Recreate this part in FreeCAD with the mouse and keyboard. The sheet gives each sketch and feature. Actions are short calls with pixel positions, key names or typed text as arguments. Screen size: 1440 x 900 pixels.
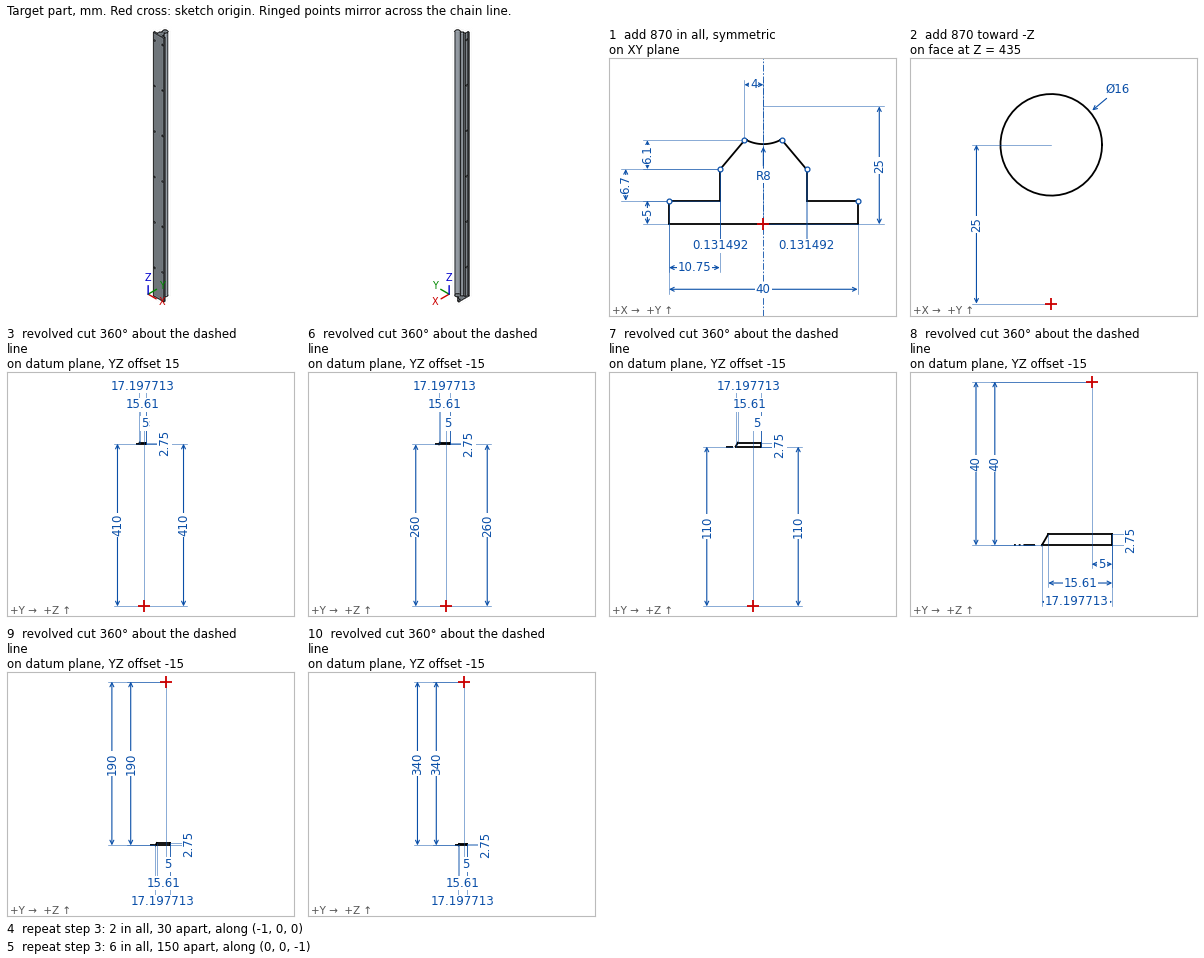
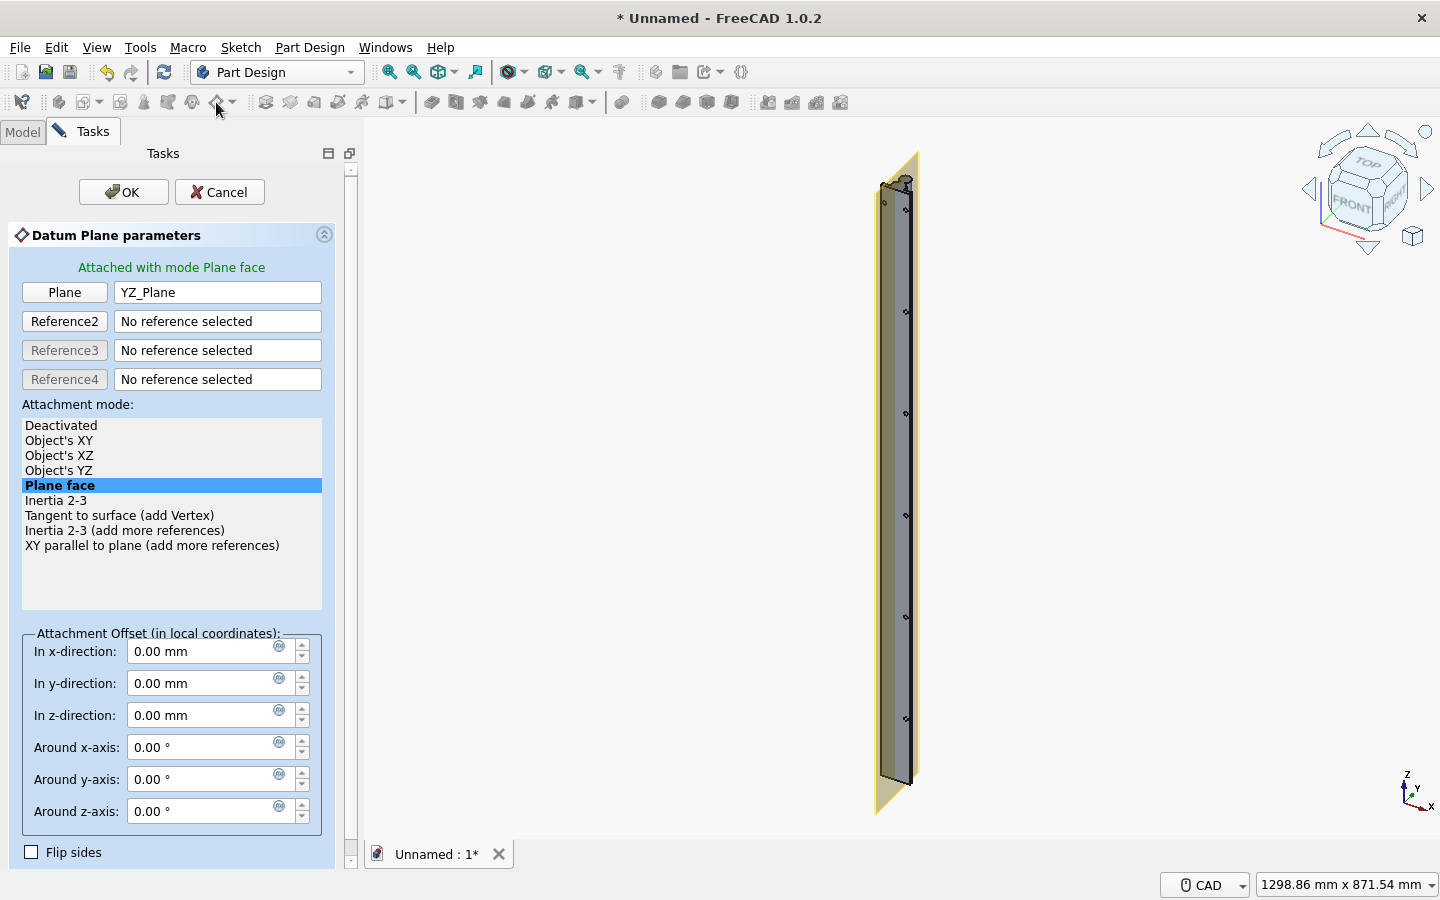
triple_click(210, 715)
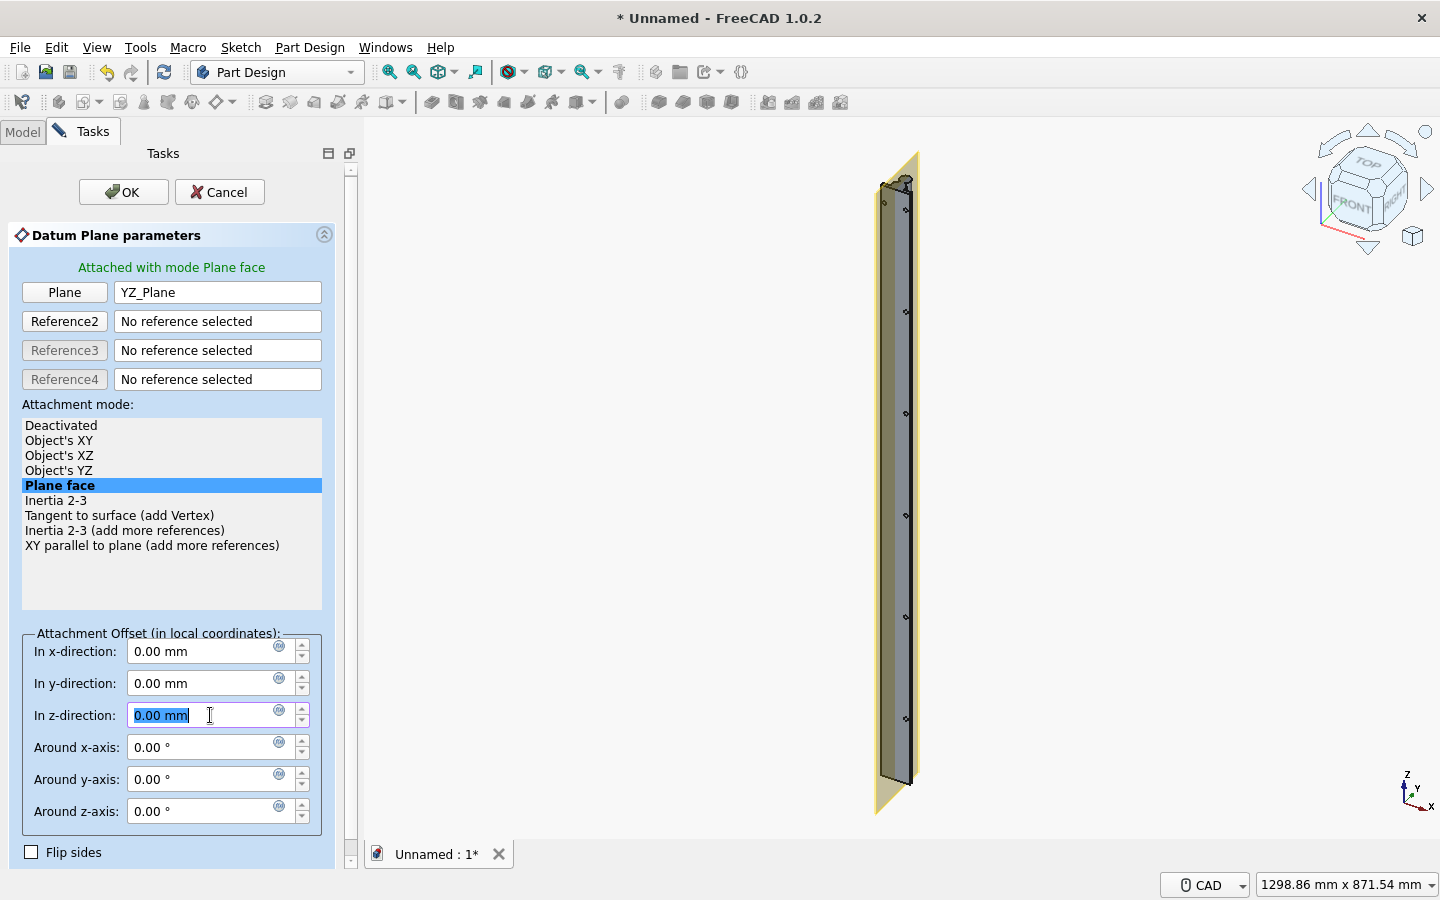
text(-15)
key(Tab)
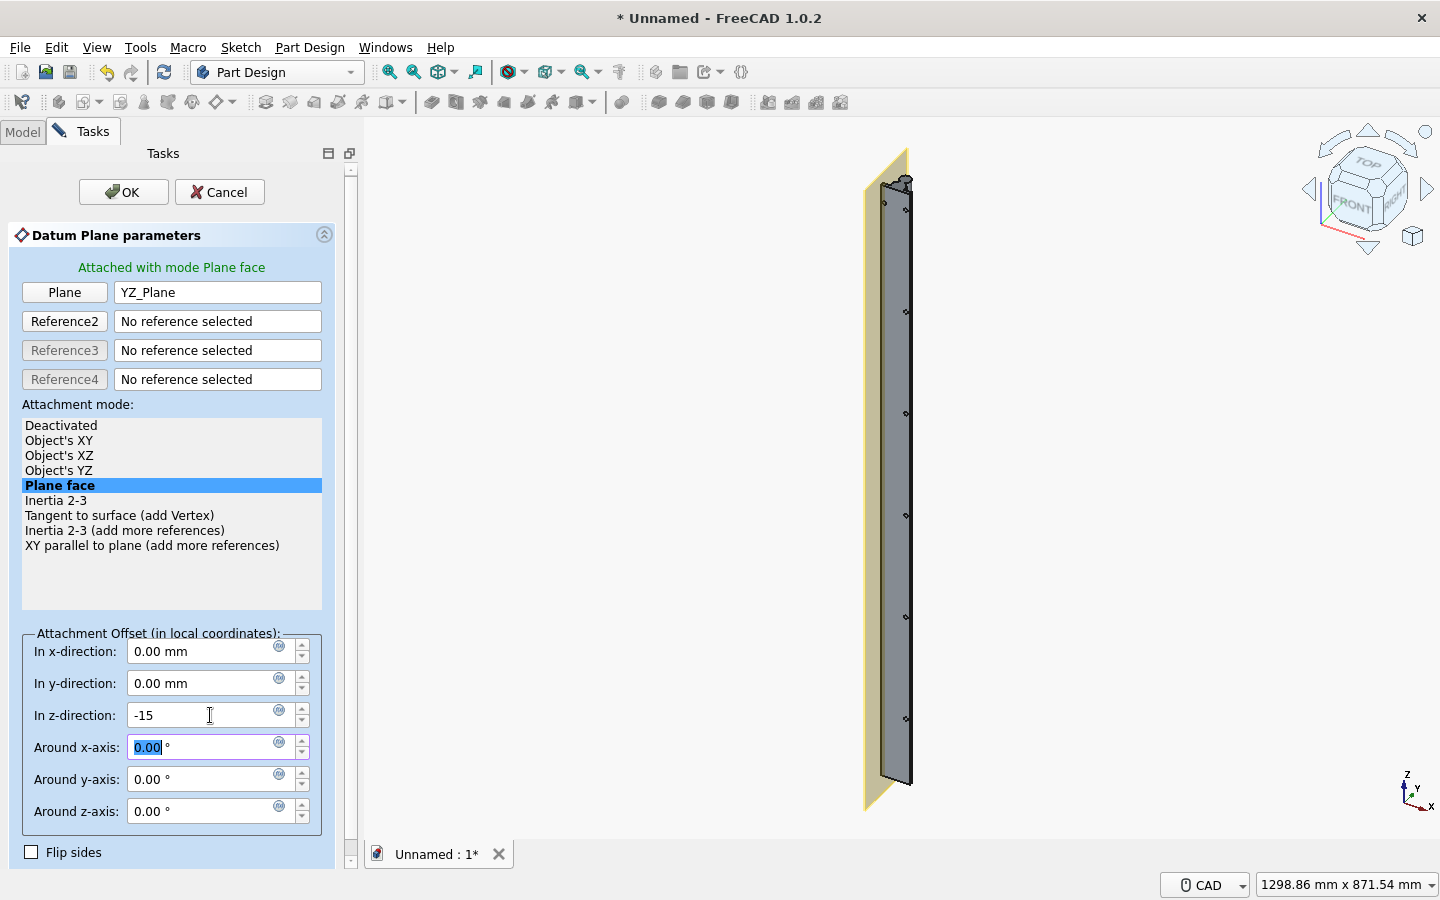
click(124, 192)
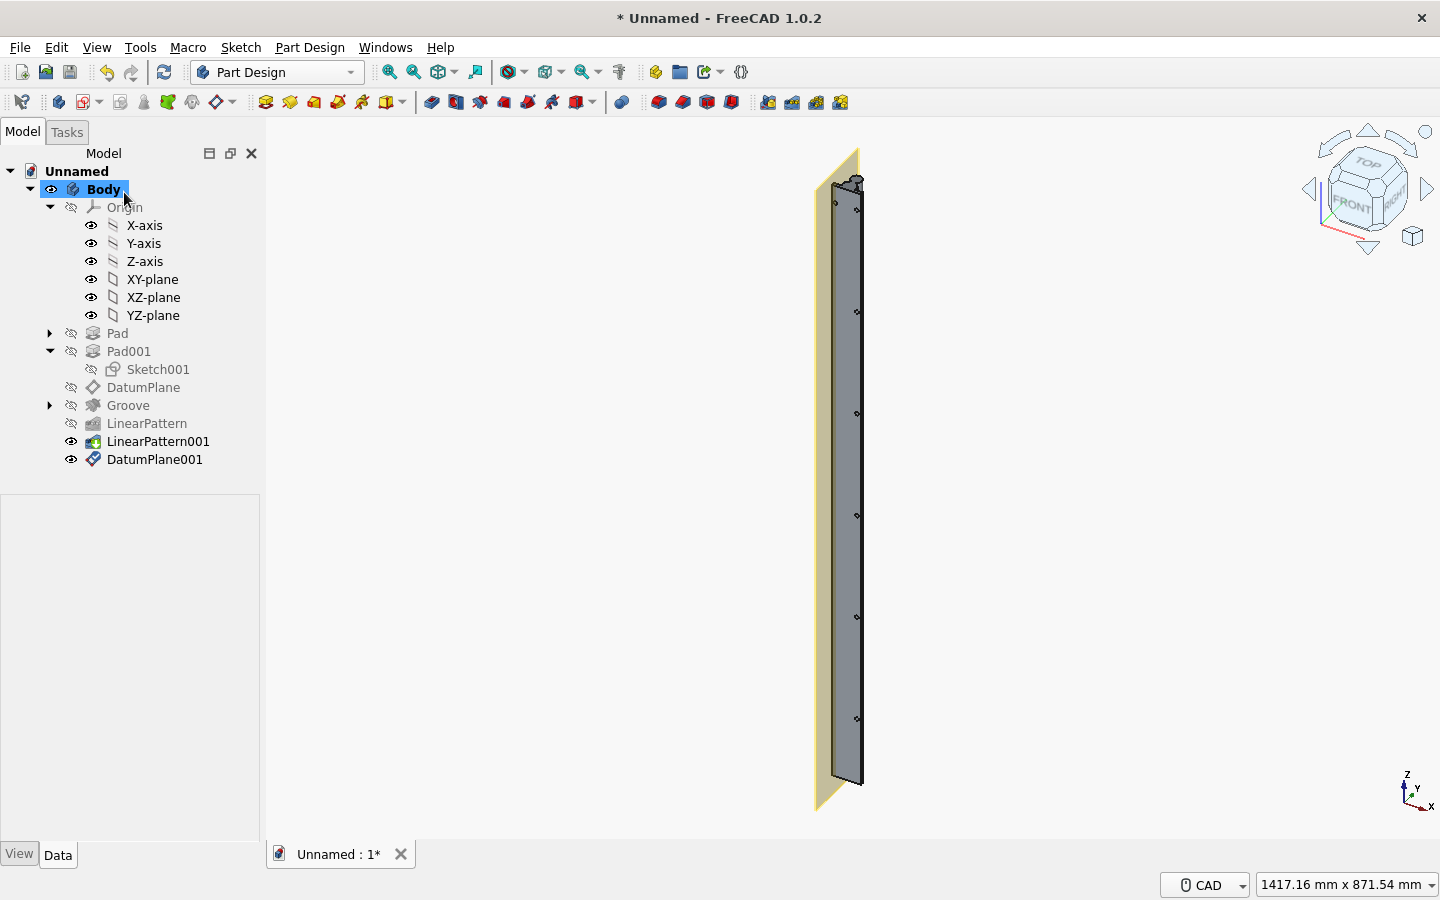
click(116, 459)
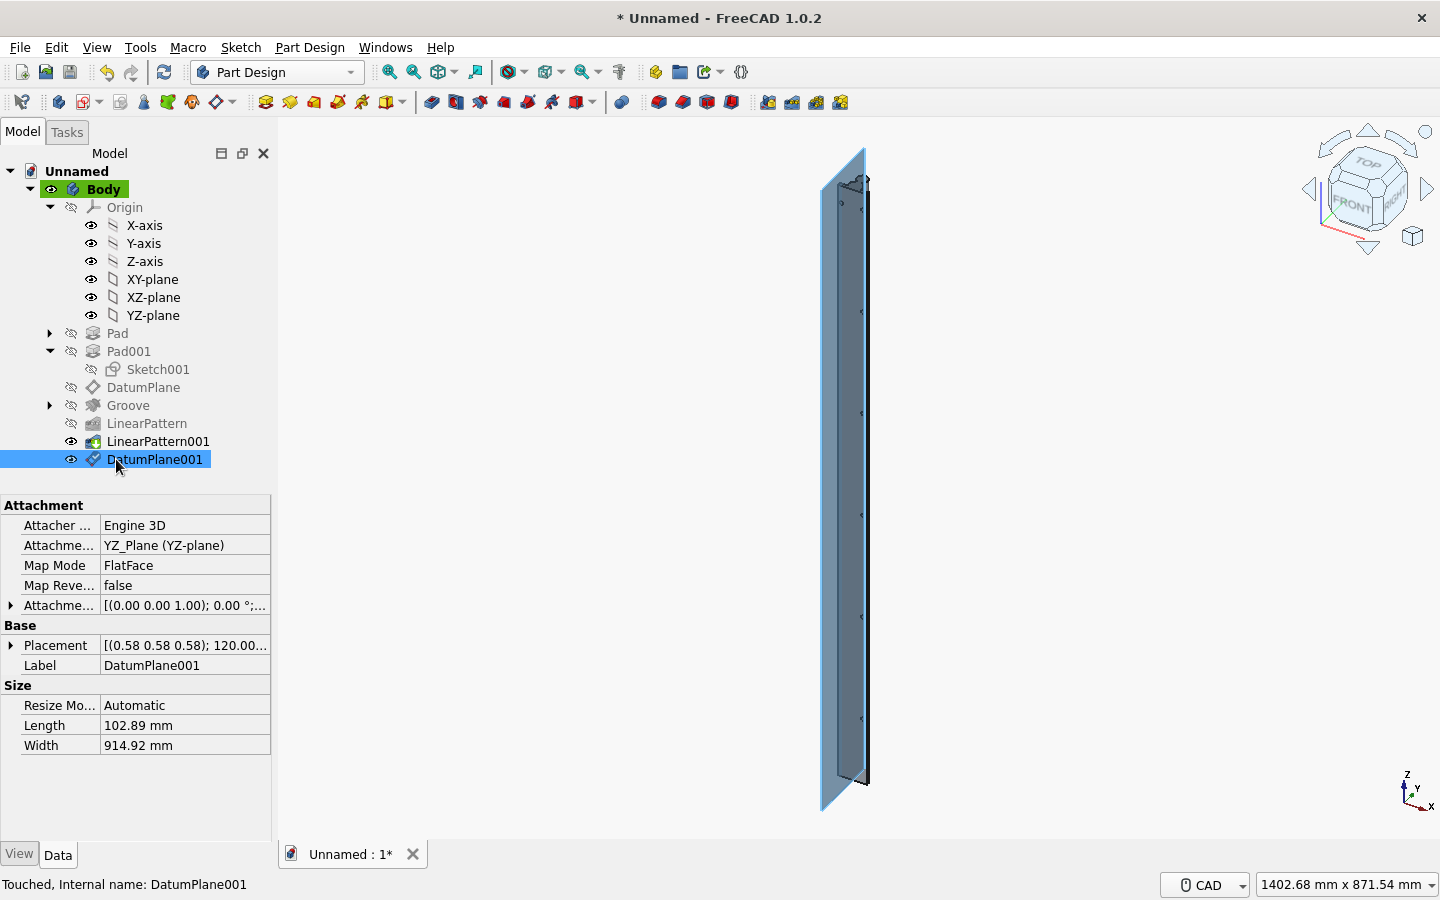
click(84, 102)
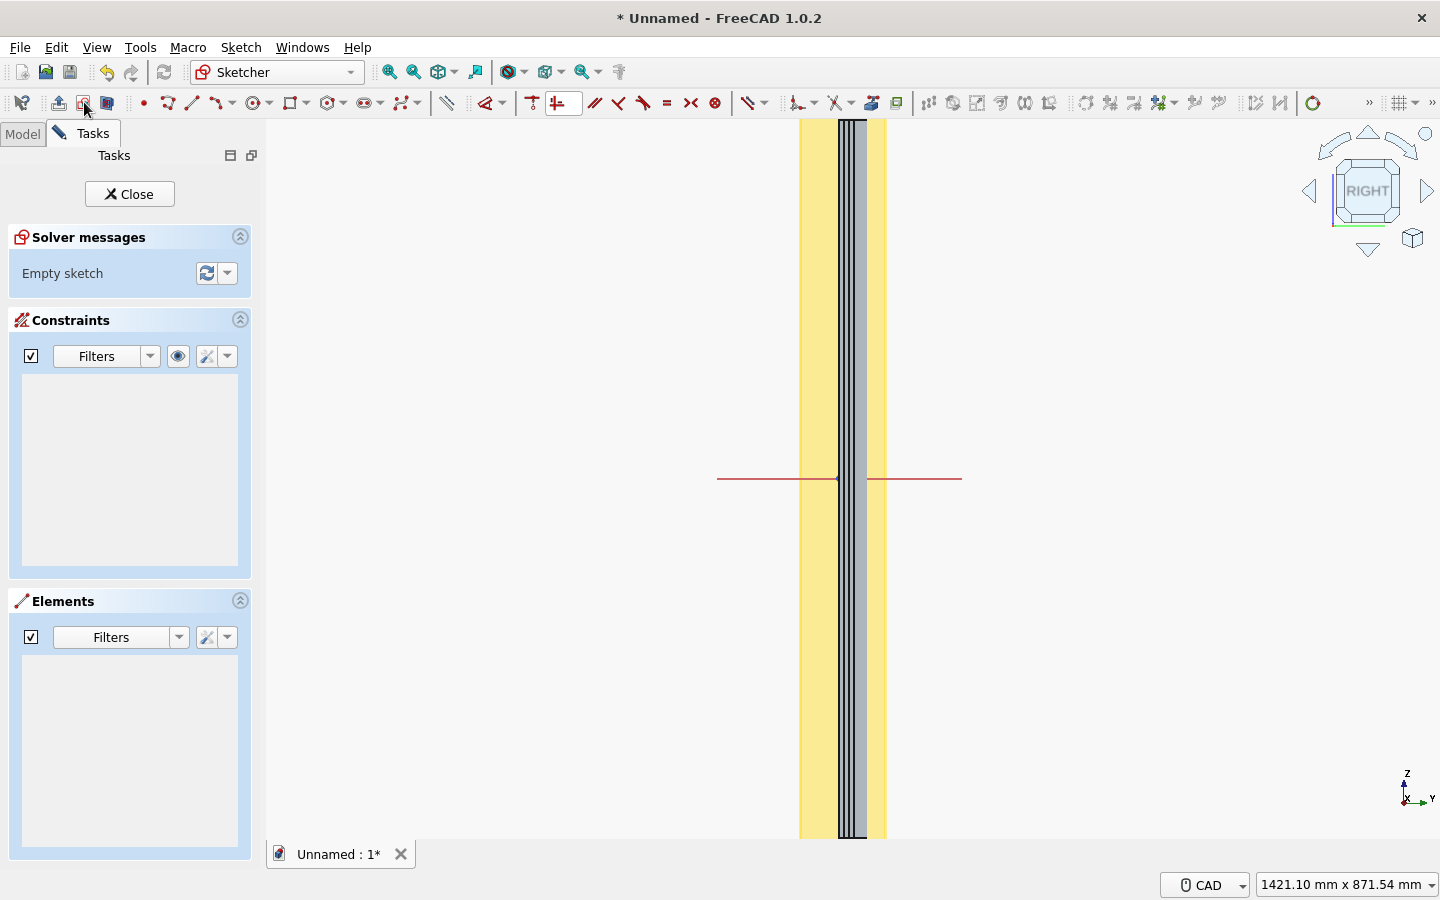
click(108, 104)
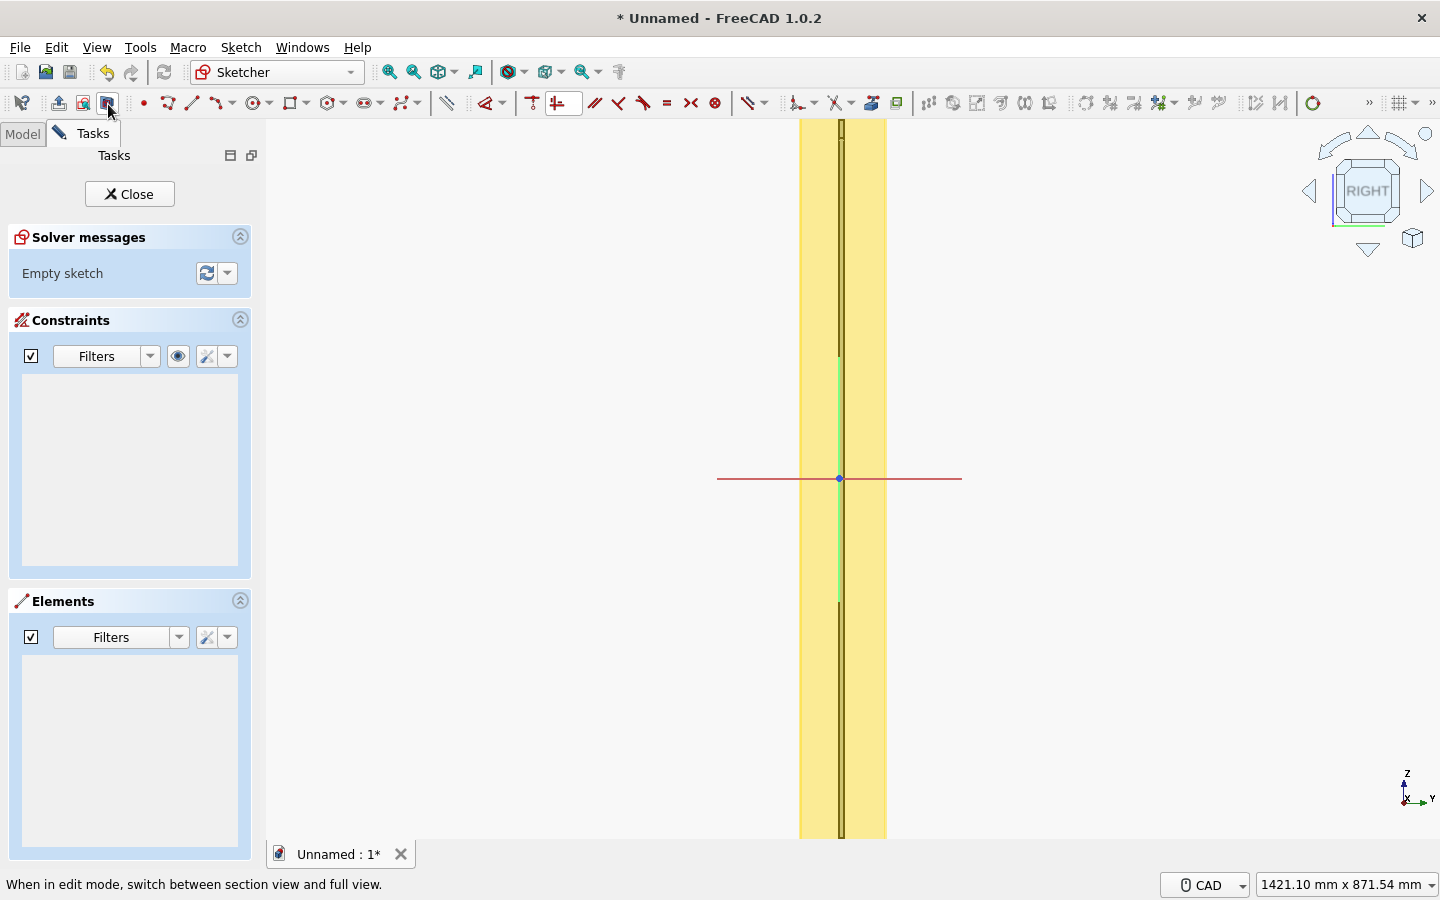
scroll(836, 252, up, 15)